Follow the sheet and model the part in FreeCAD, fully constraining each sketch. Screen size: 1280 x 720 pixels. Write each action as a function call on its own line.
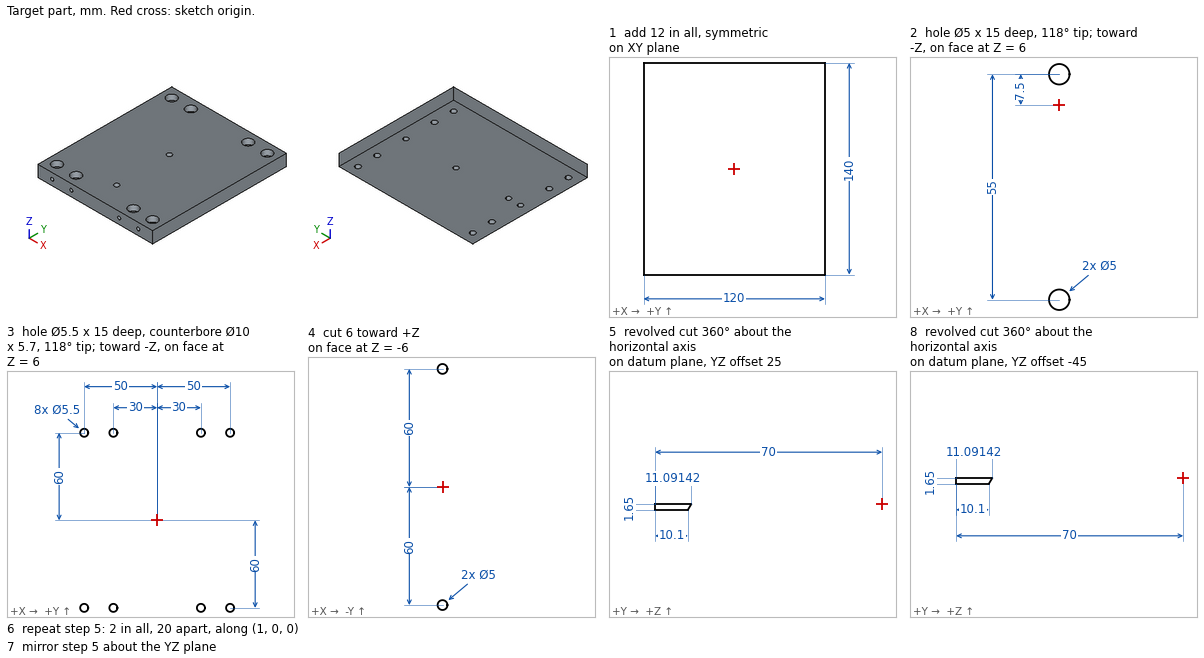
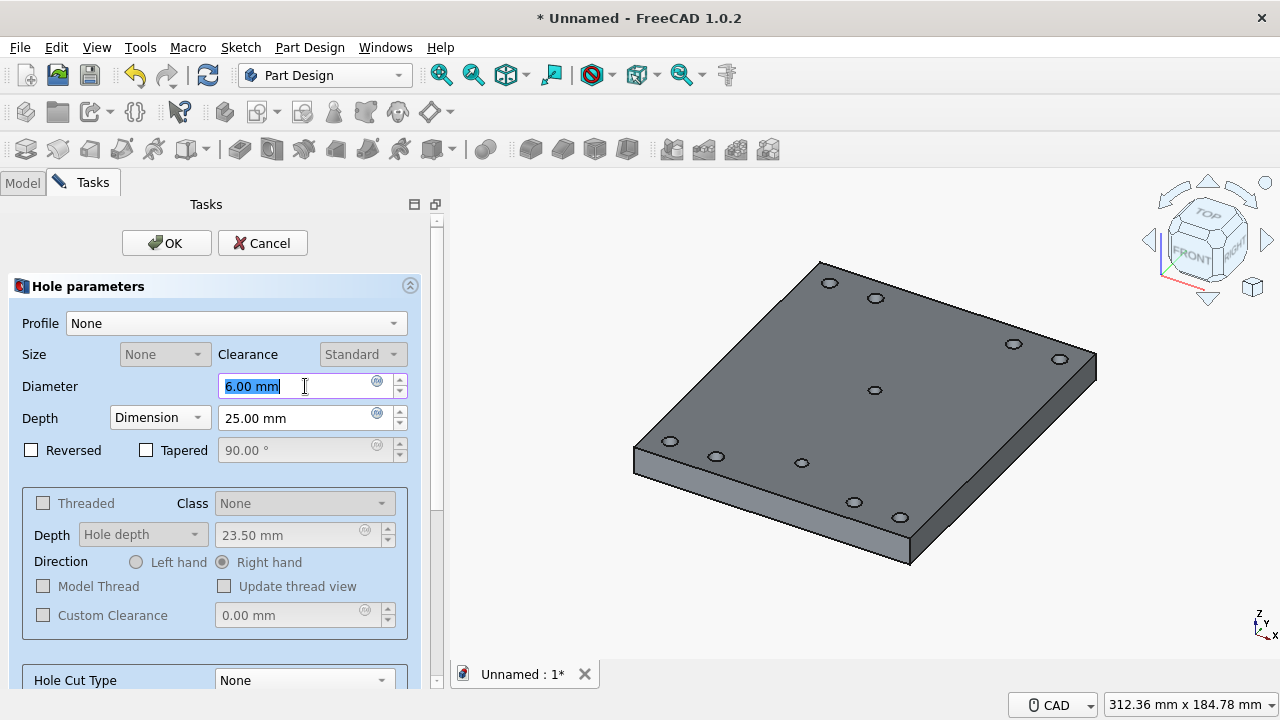
text(5.5)
key(Tab)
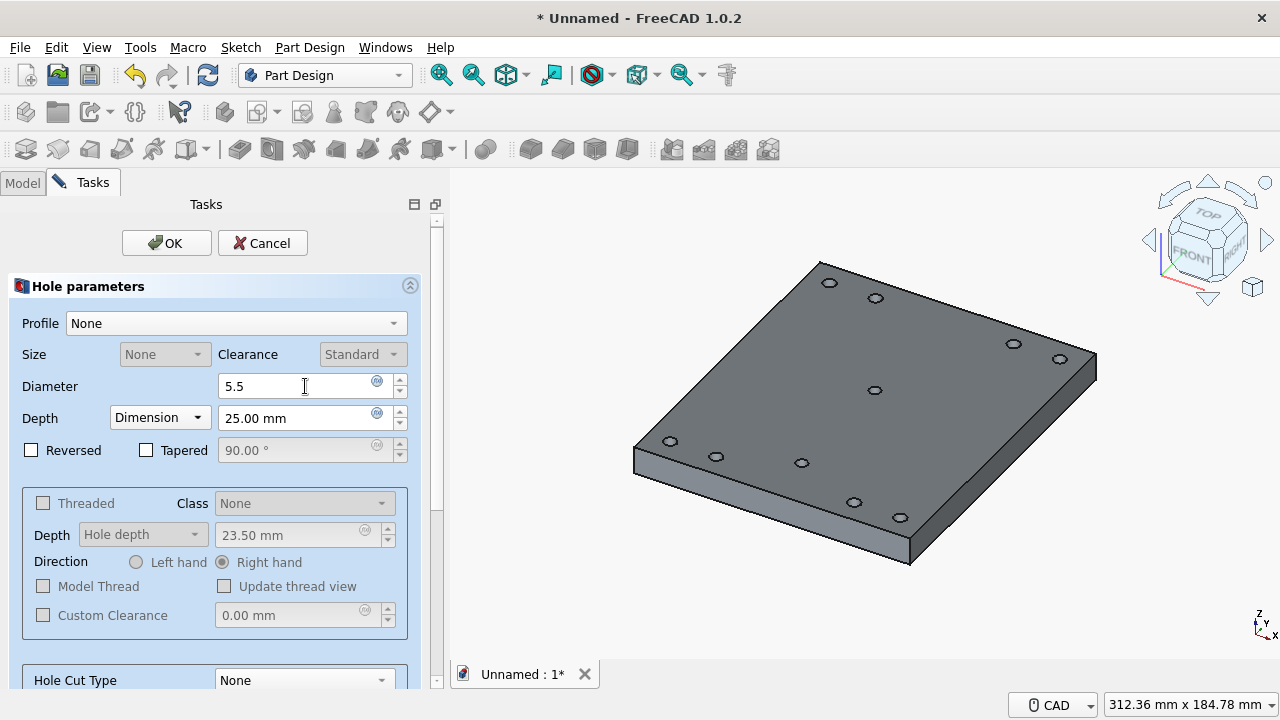
triple_click(305, 418)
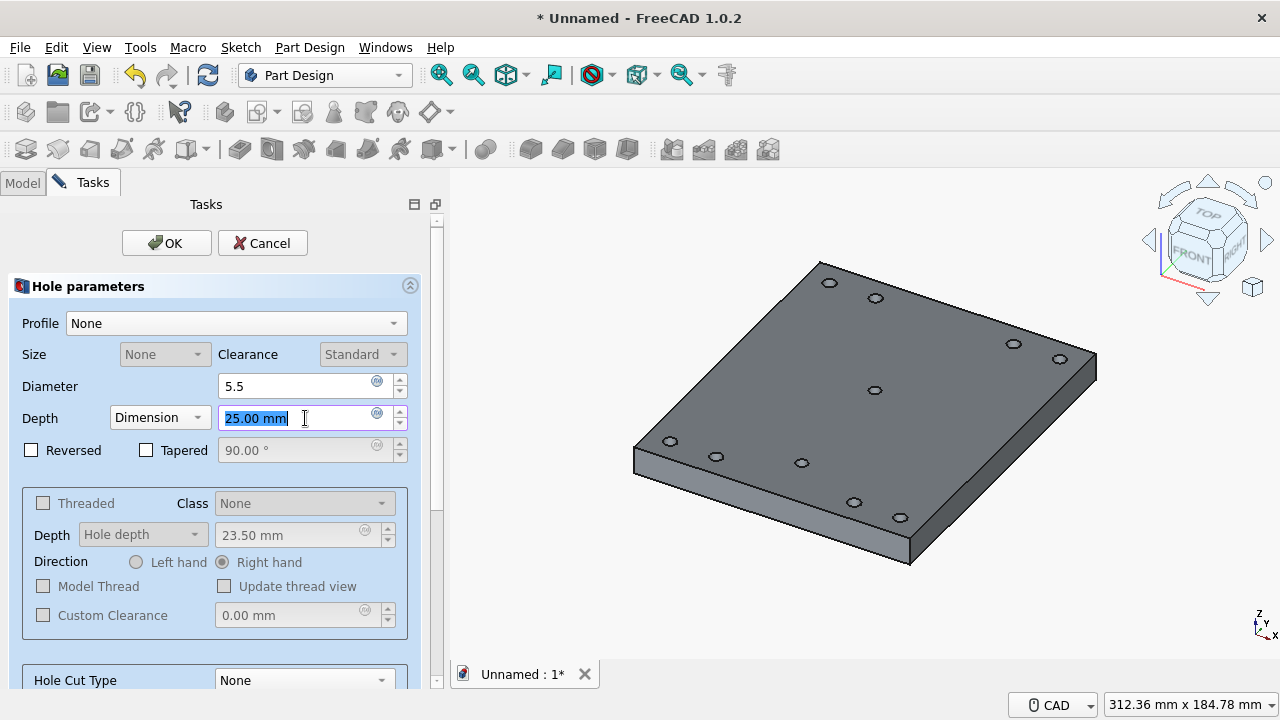
text(15)
key(Tab)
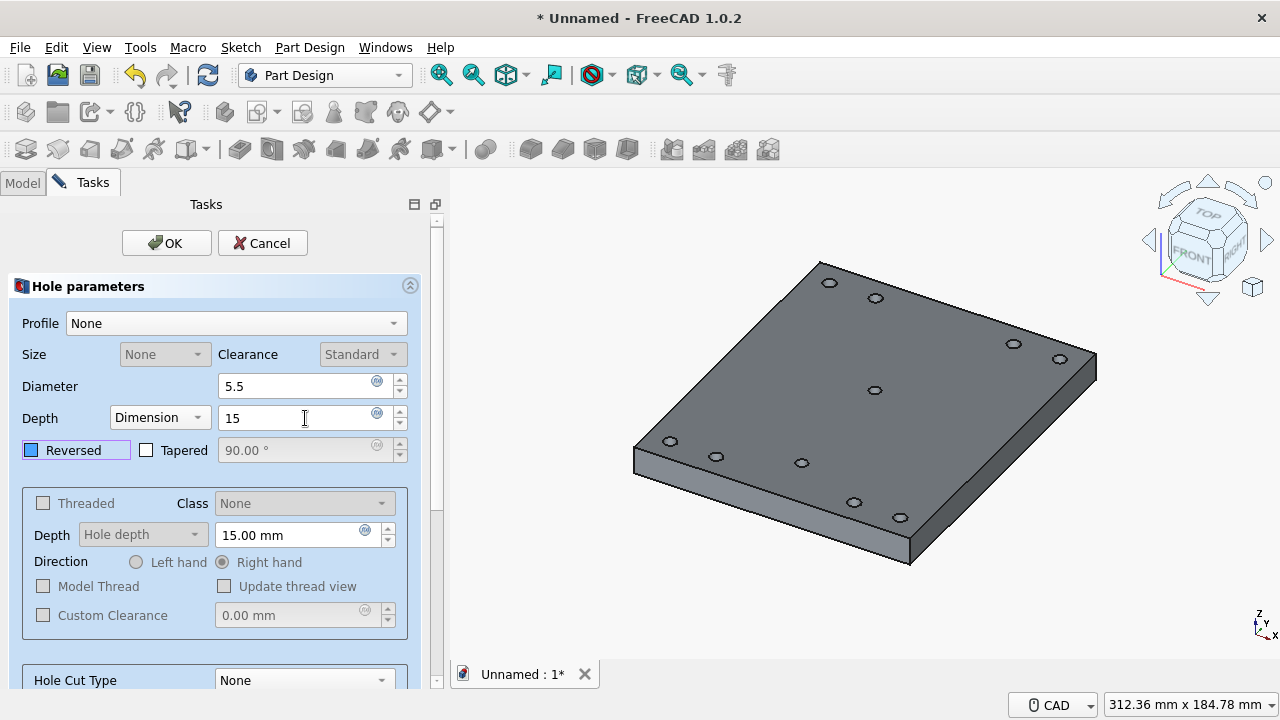
scroll(437, 451, down, 2)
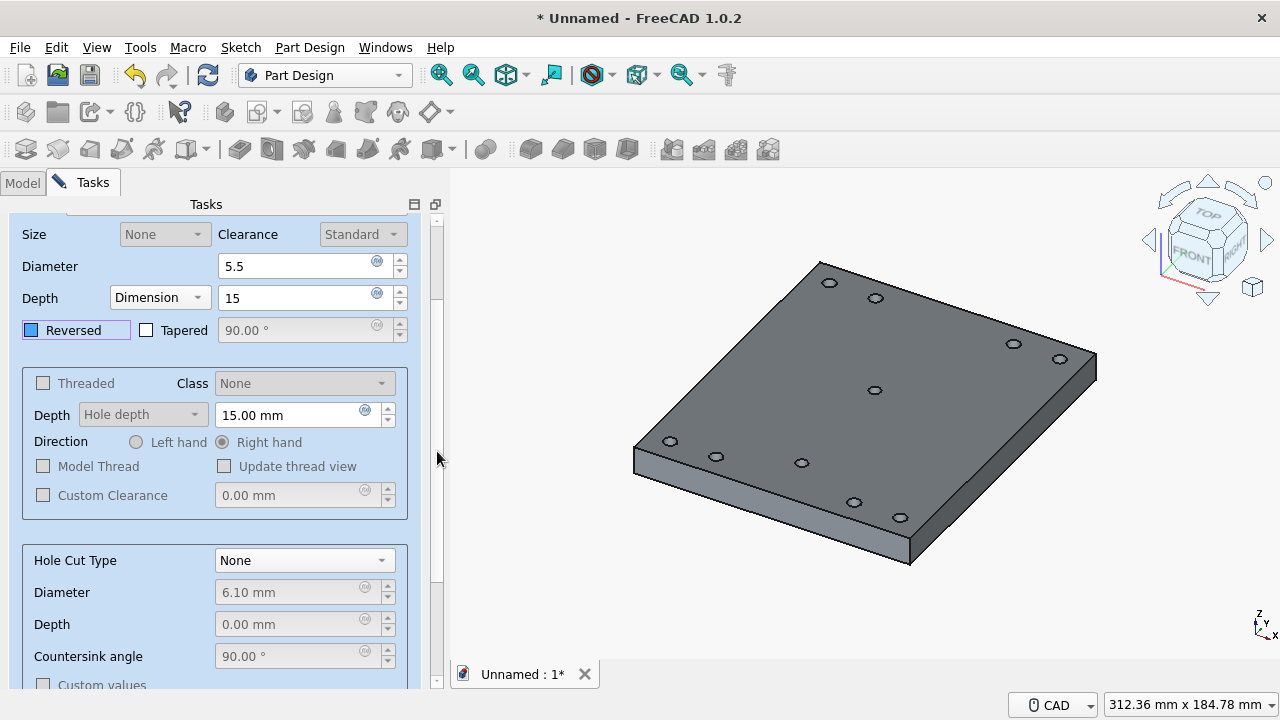
click(306, 560)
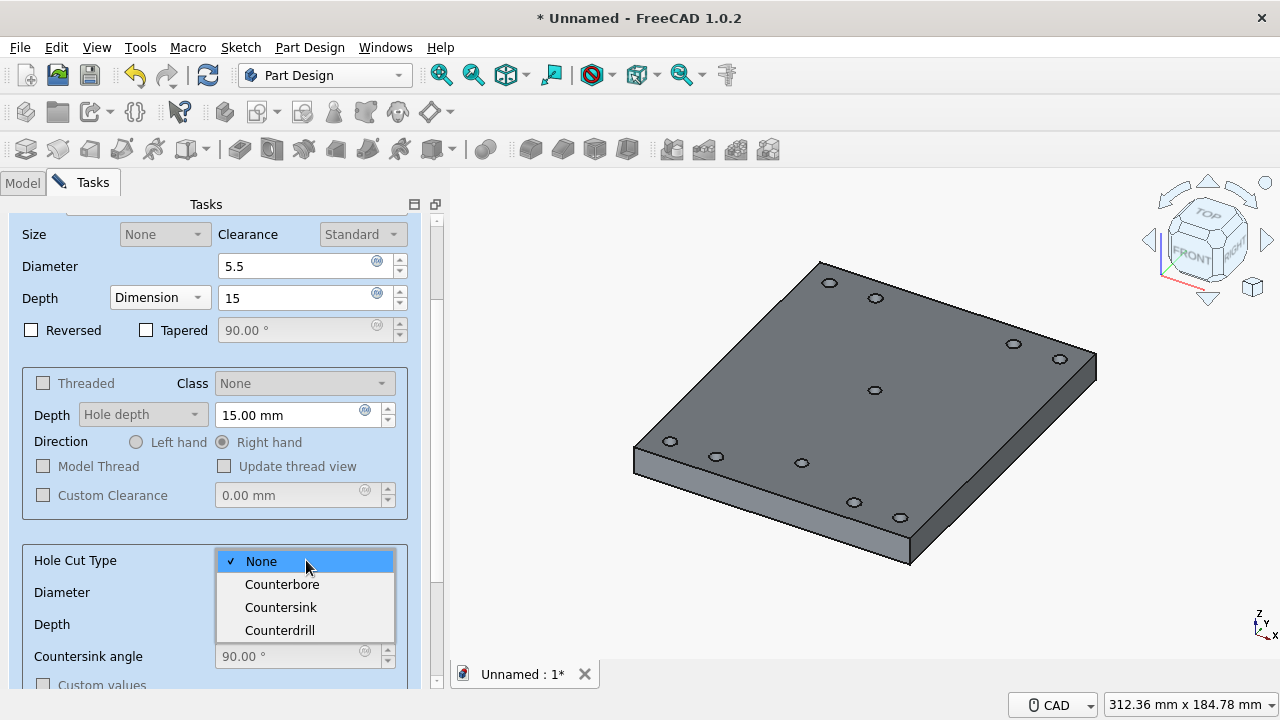
click(304, 584)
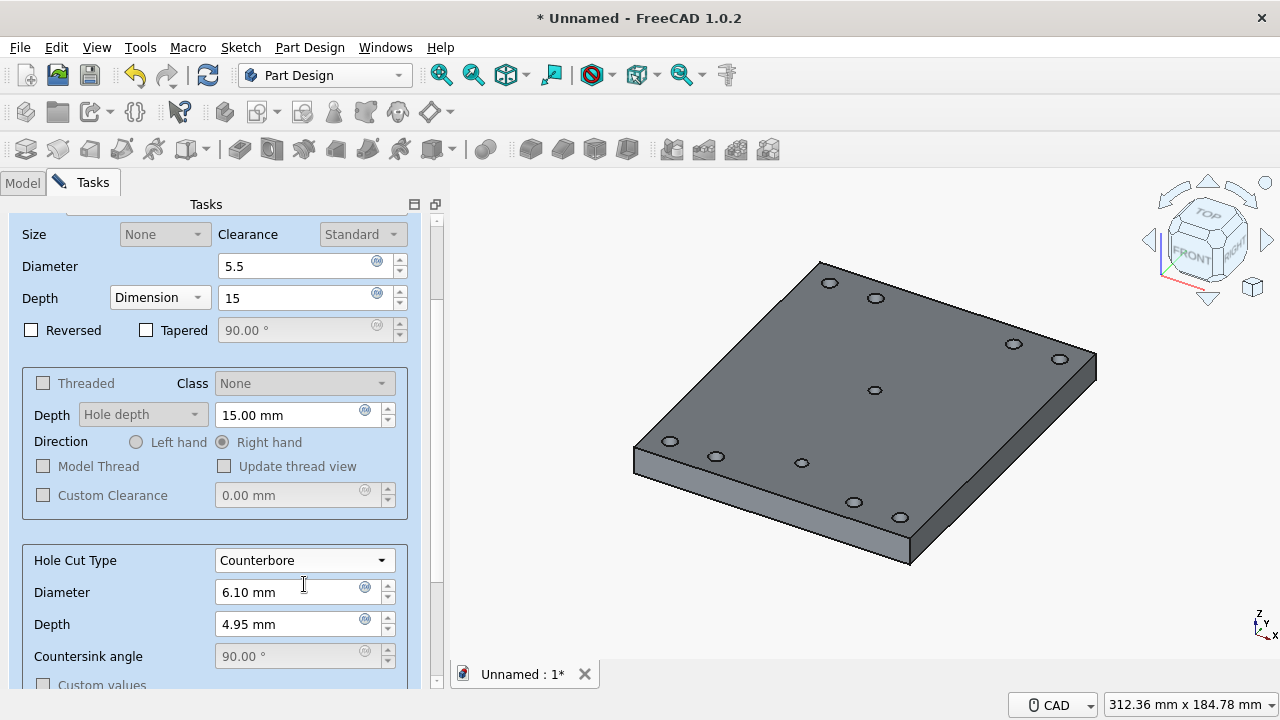
triple_click(298, 592)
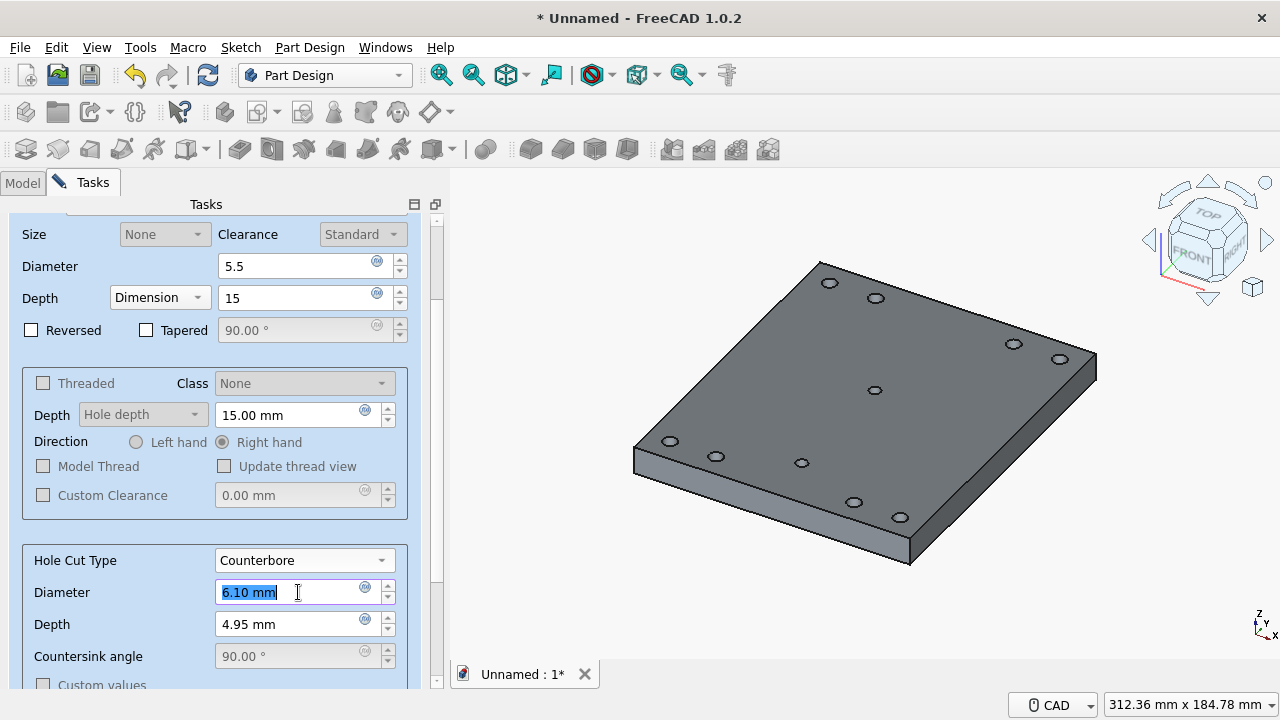
text(10)
key(Tab)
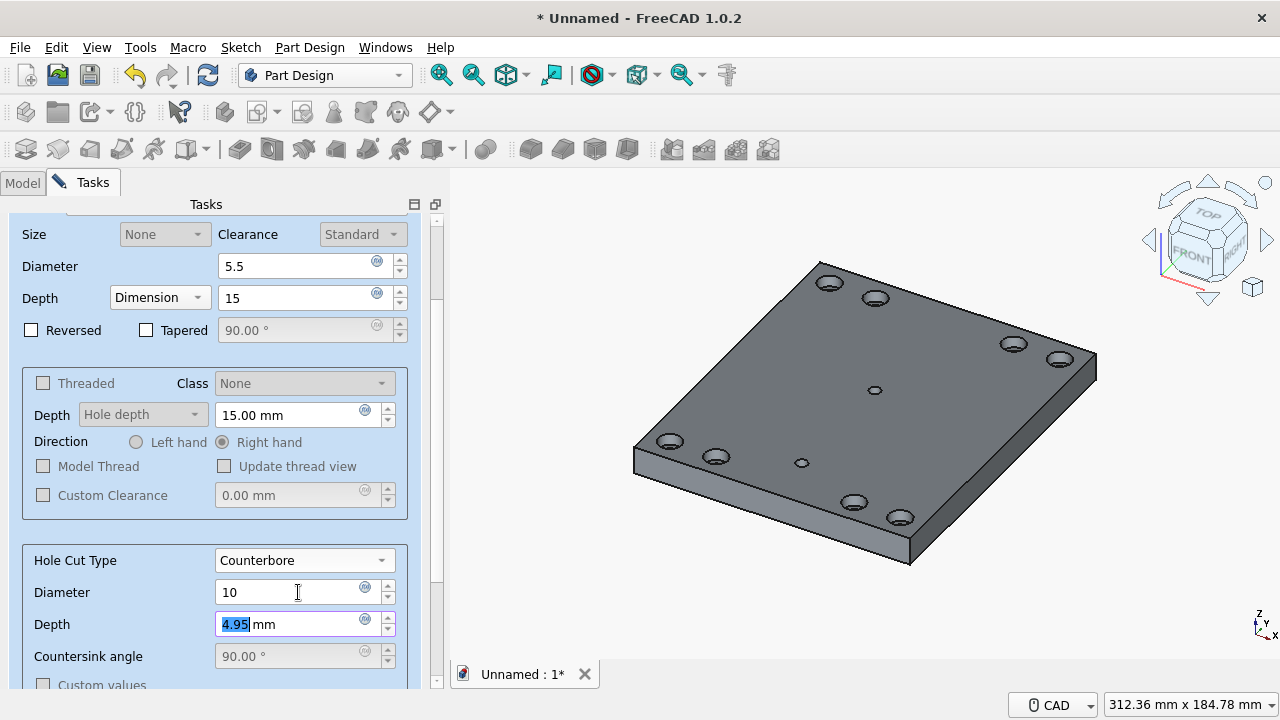
text(5.7)
key(Tab)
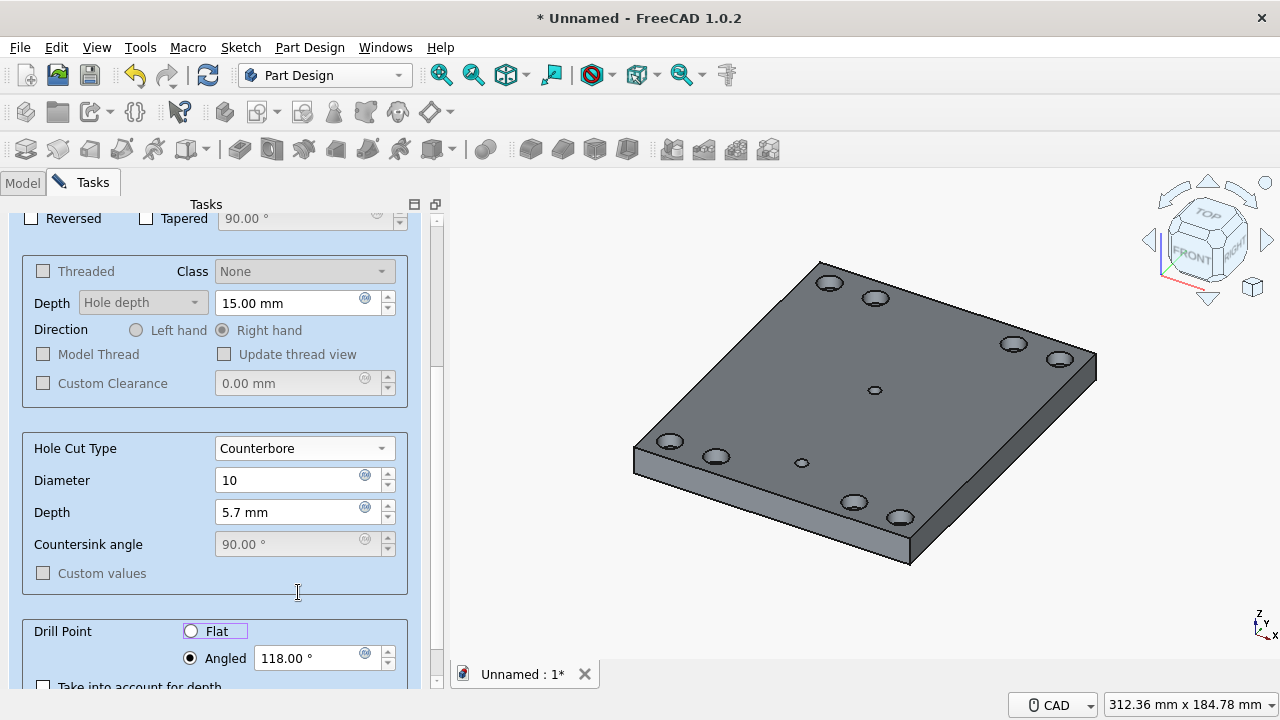
scroll(437, 451, up, 5)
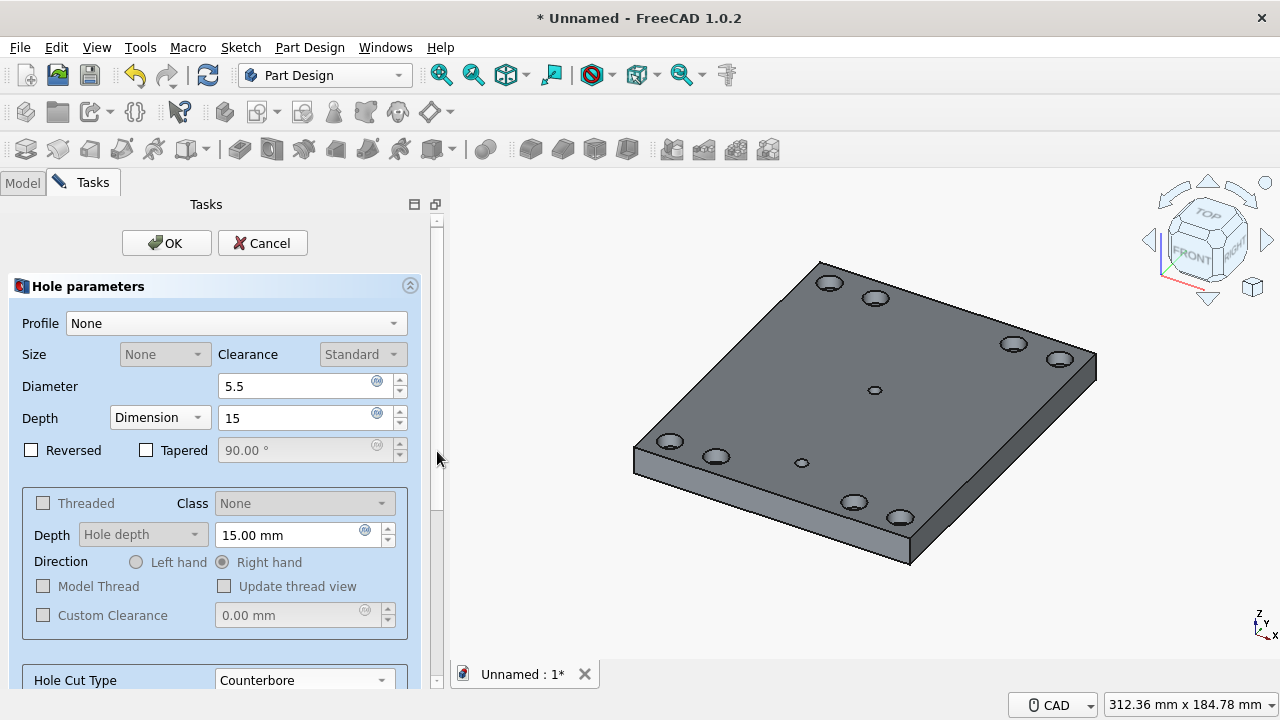
click(167, 243)